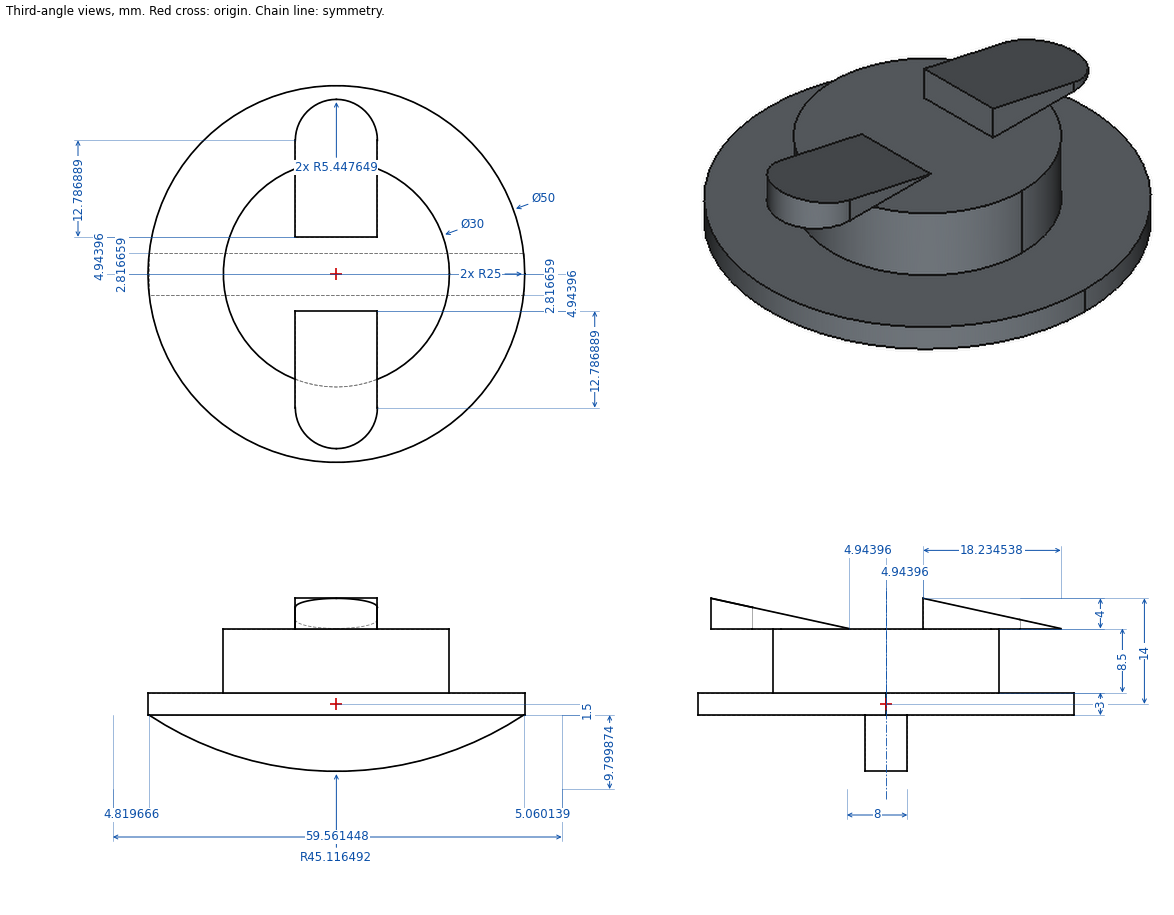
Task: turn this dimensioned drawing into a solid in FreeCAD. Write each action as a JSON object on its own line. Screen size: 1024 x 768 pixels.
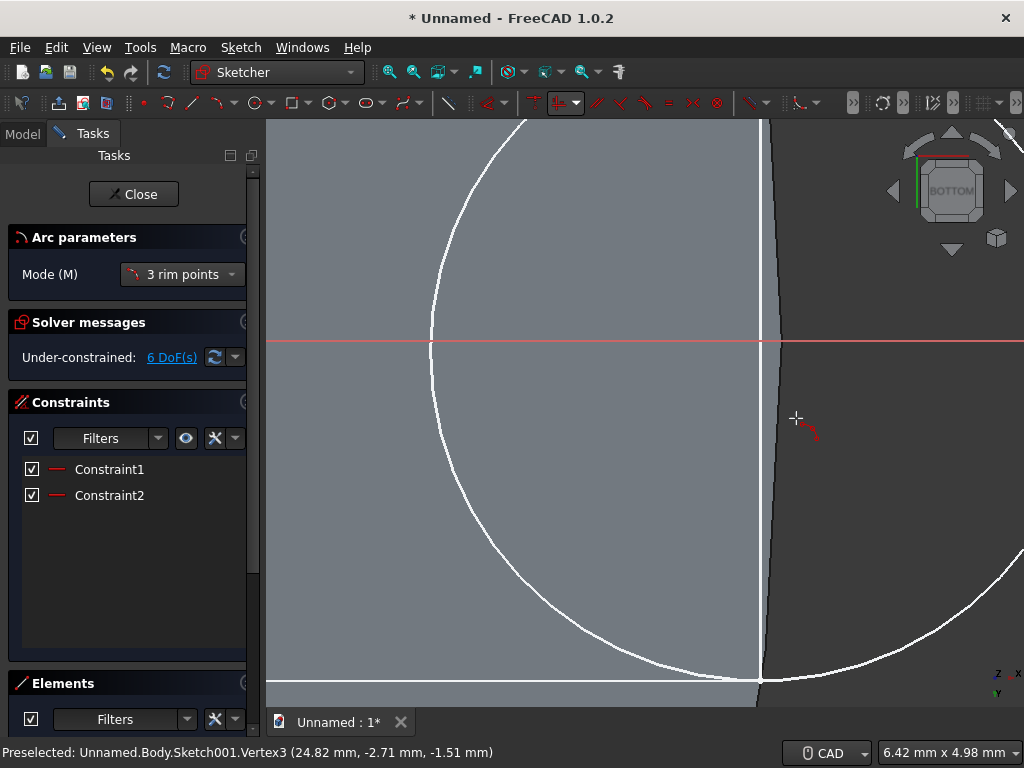
{"action": "left_click", "coordinate": [781, 408]}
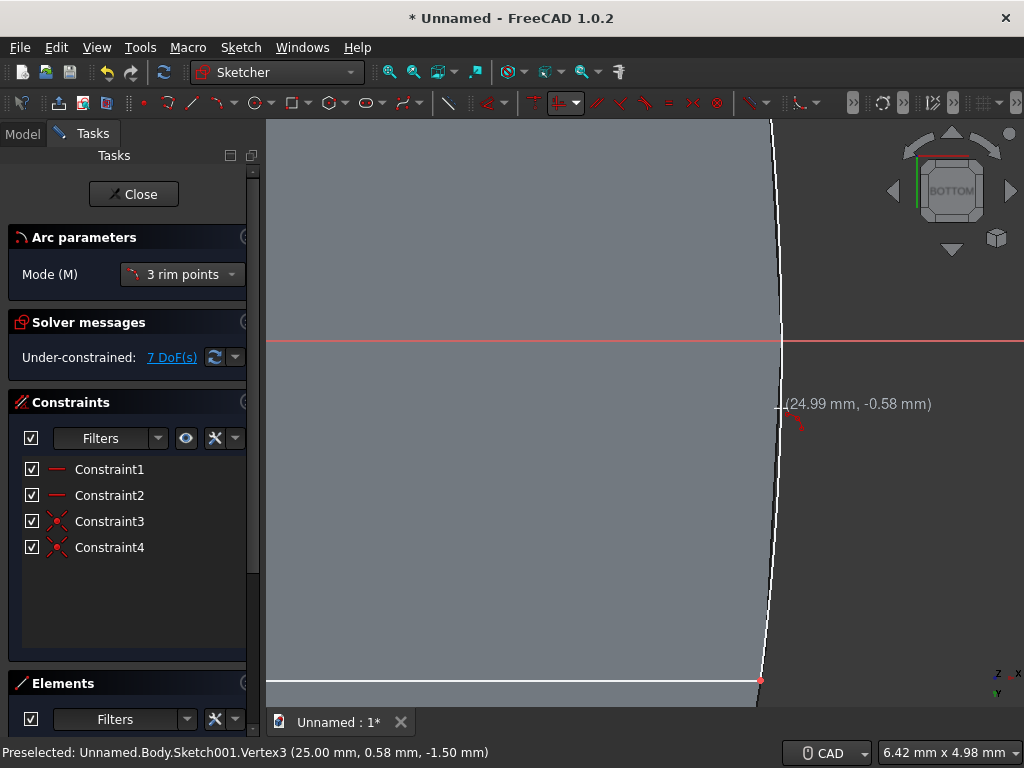
{"action": "scroll", "coordinate": [797, 419], "scroll_direction": "down", "scroll_amount": 13}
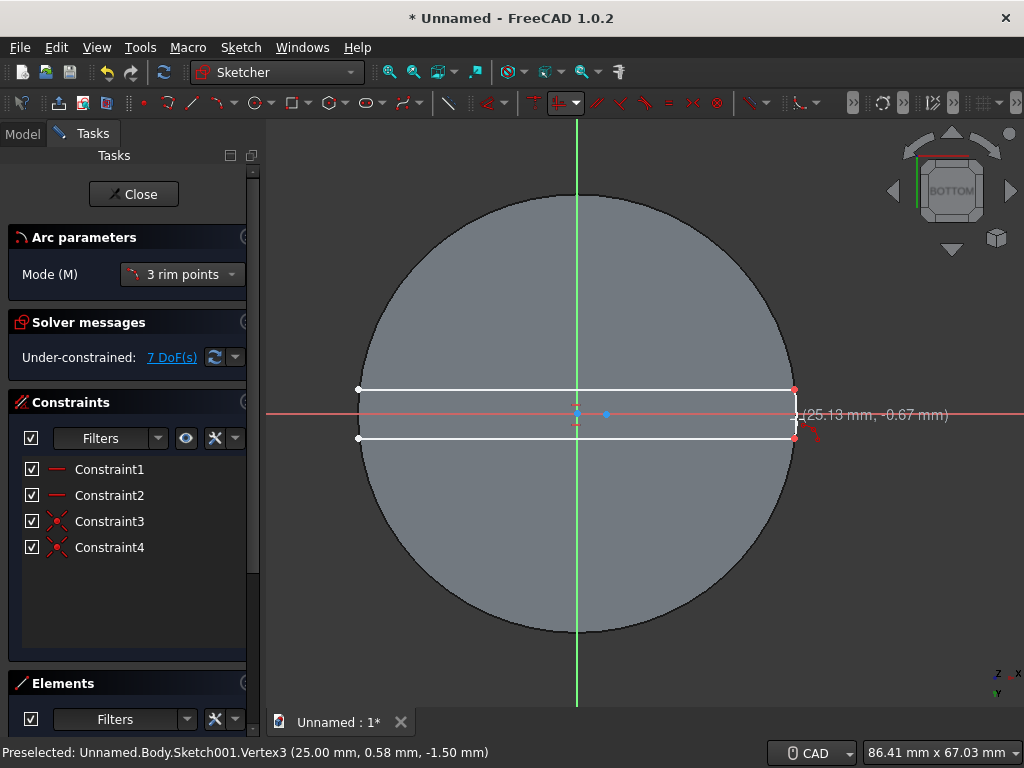
{"action": "left_click", "coordinate": [359, 390]}
{"action": "left_click", "coordinate": [359, 439]}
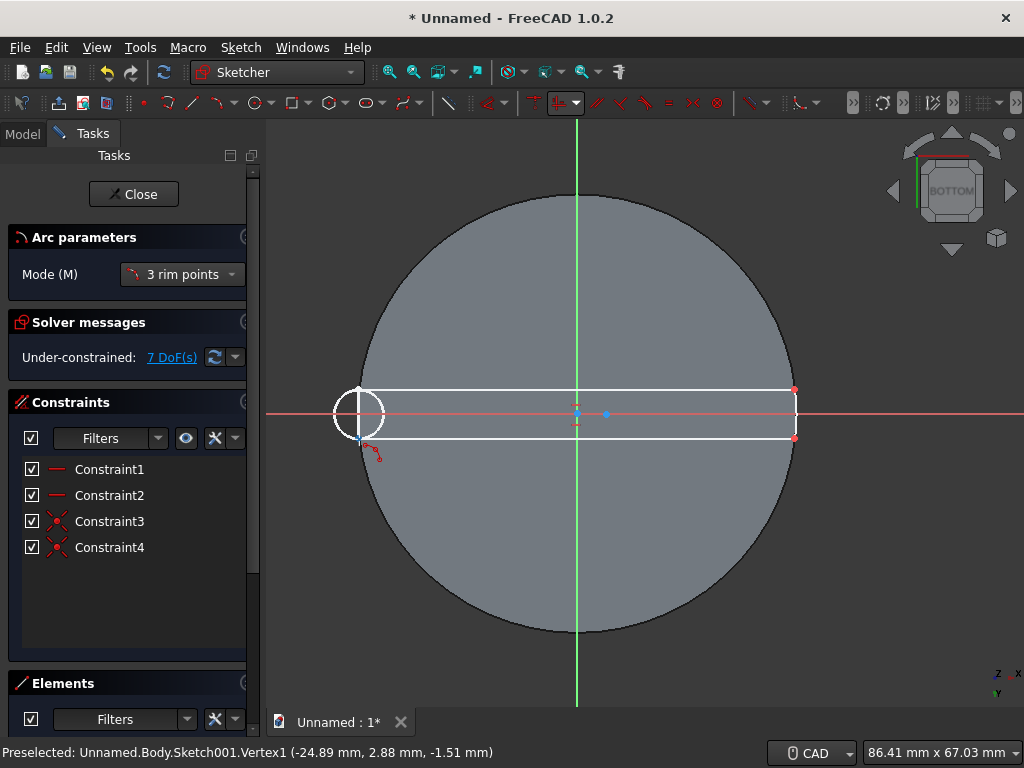
{"action": "scroll", "coordinate": [358, 409], "scroll_direction": "up", "scroll_amount": 13}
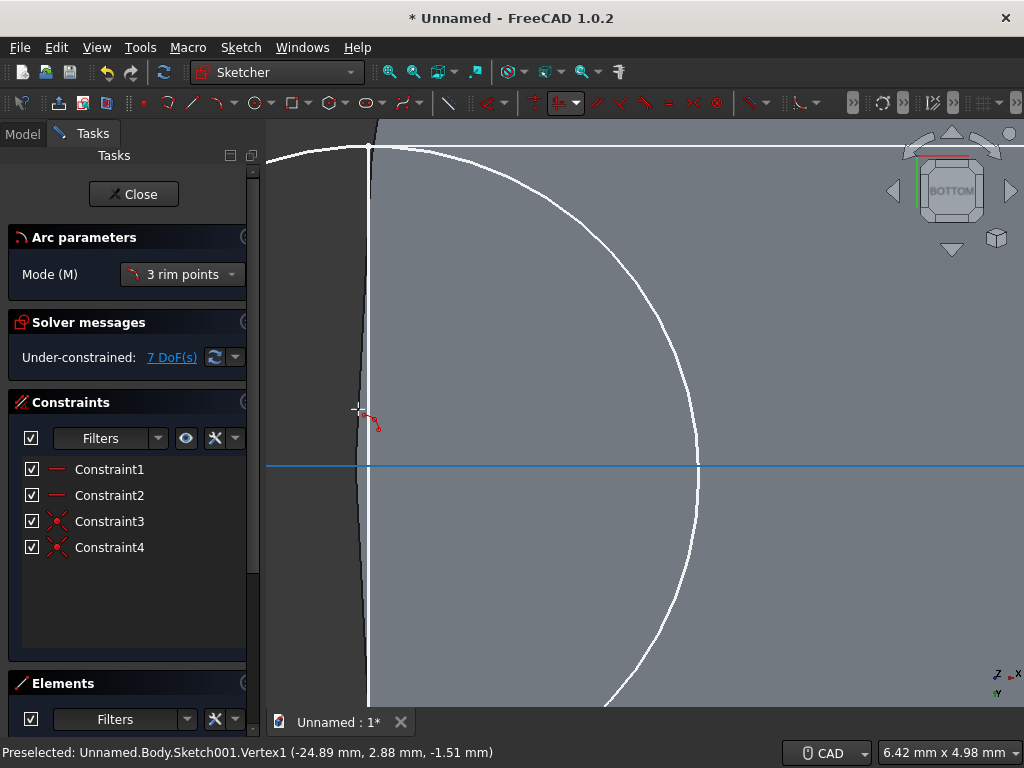
{"action": "left_click", "coordinate": [356, 399]}
{"action": "key", "text": "Escape"}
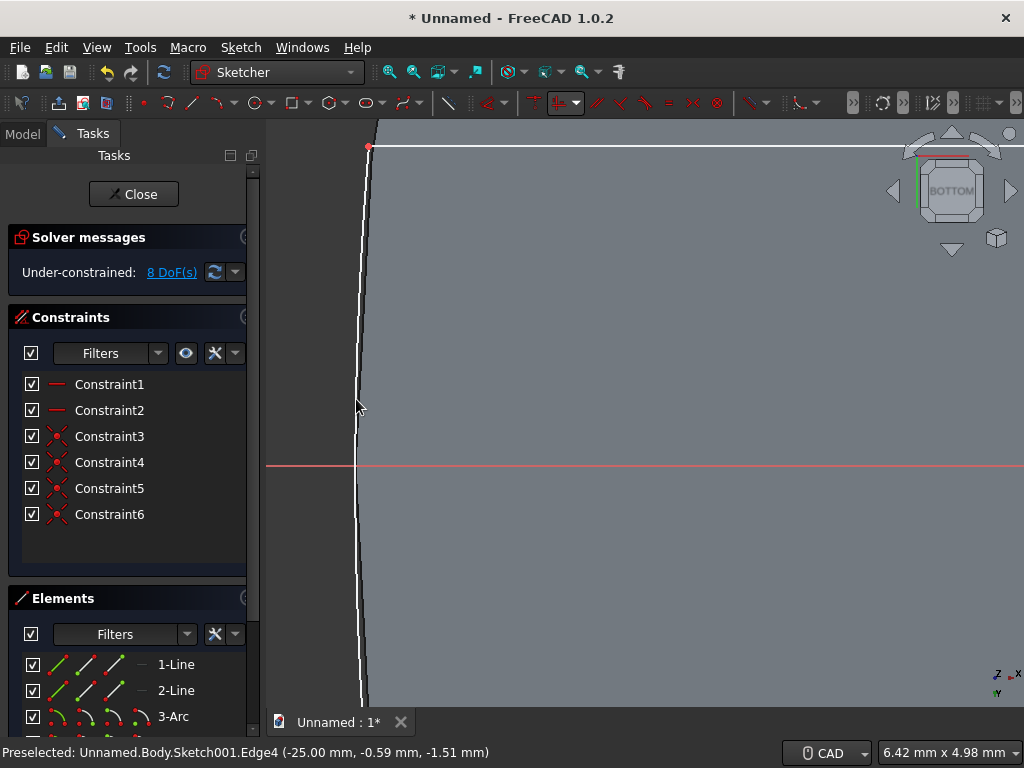
{"action": "scroll", "coordinate": [357, 409], "scroll_direction": "down", "scroll_amount": 13}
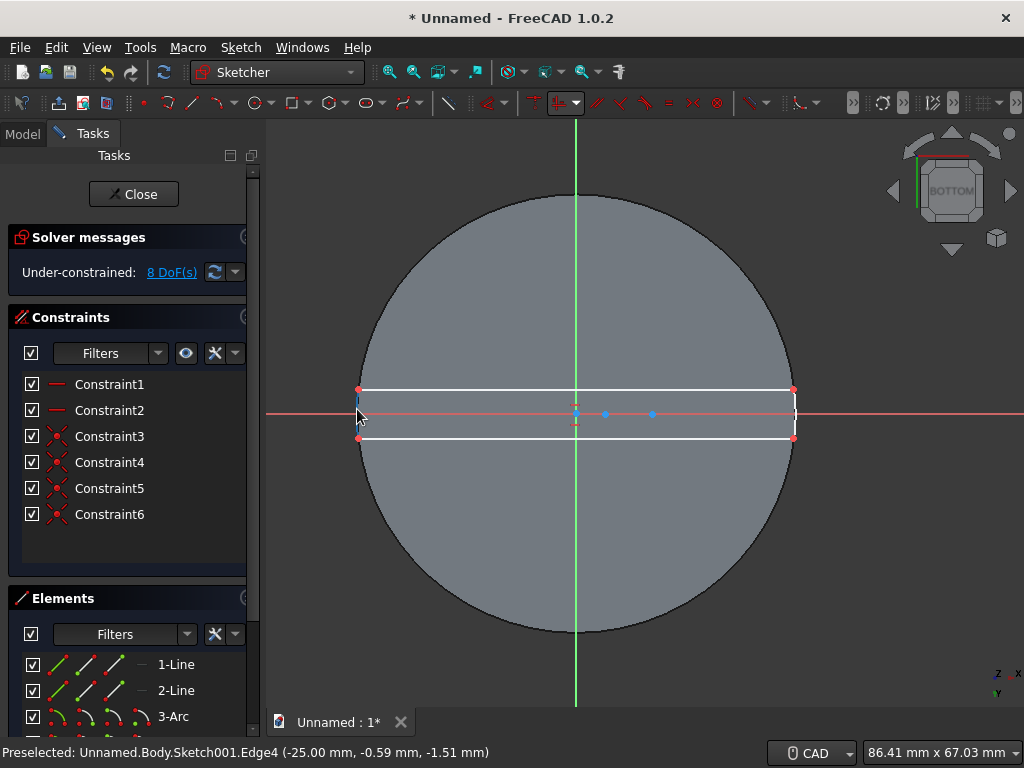
{"action": "scroll", "coordinate": [795, 424], "scroll_direction": "up", "scroll_amount": 2}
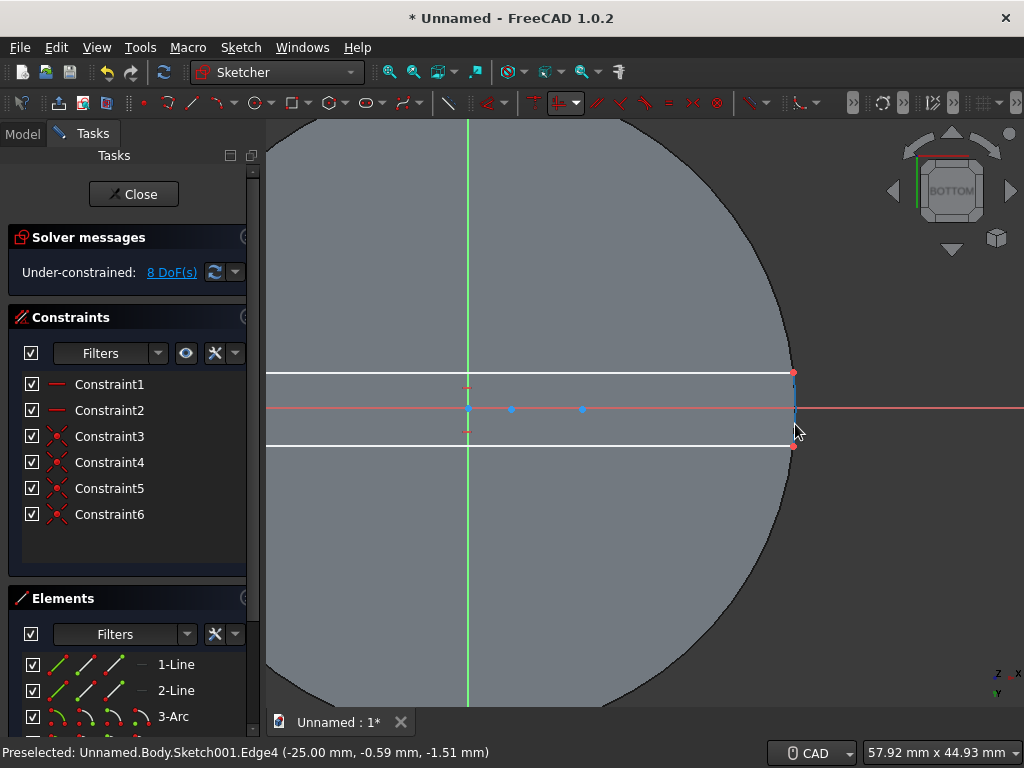
{"action": "left_click", "coordinate": [795, 424]}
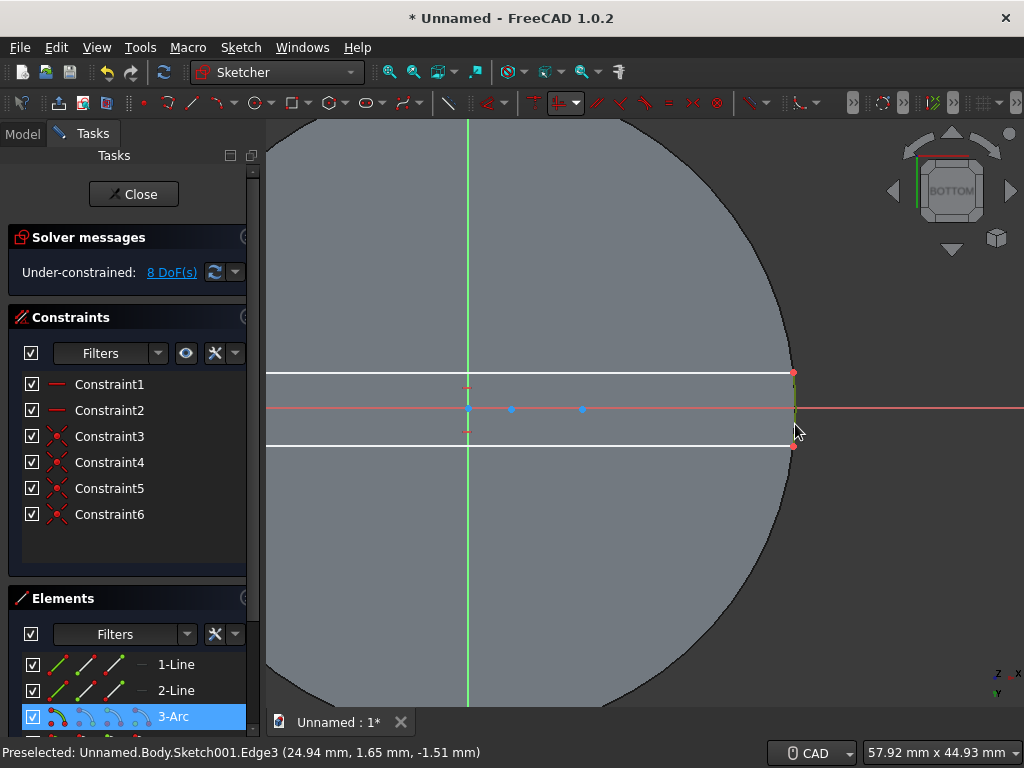
{"action": "scroll", "coordinate": [796, 422], "scroll_direction": "down", "scroll_amount": 2}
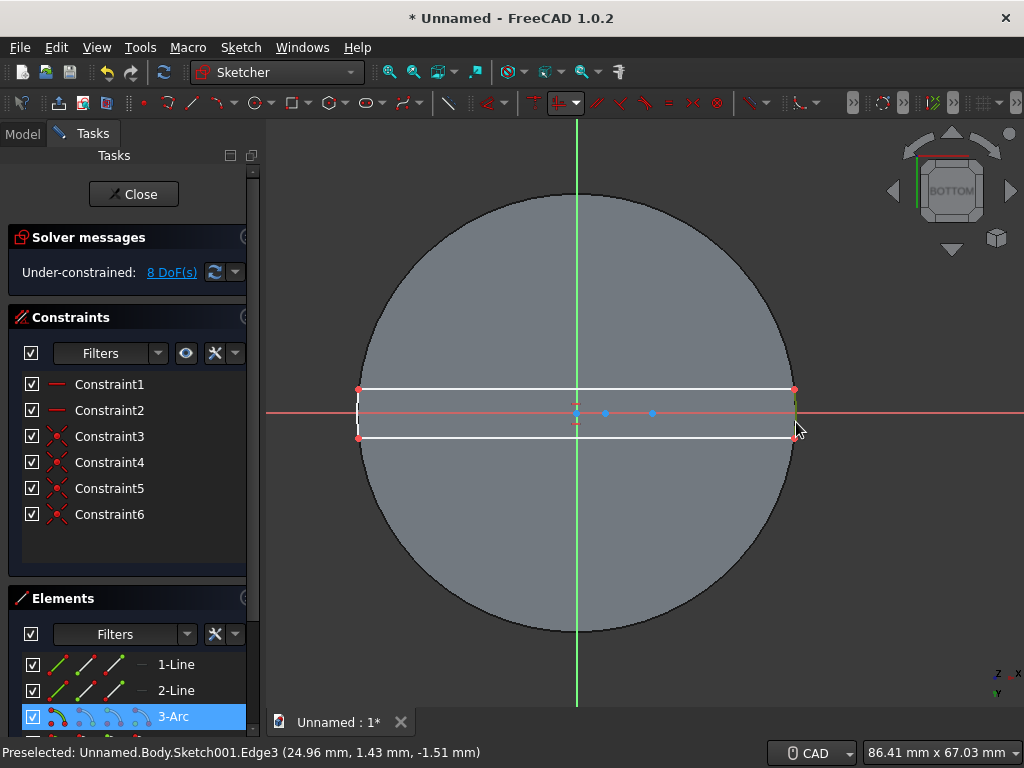
{"action": "scroll", "coordinate": [357, 404], "scroll_direction": "up", "scroll_amount": 3}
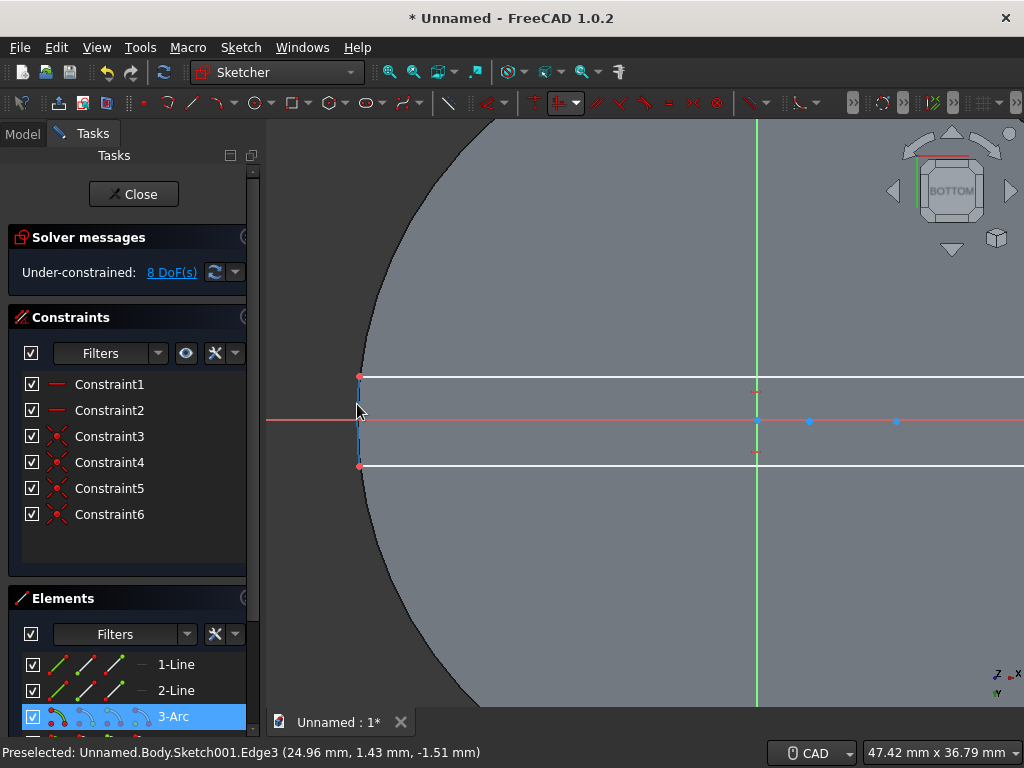
{"action": "left_click", "coordinate": [358, 404]}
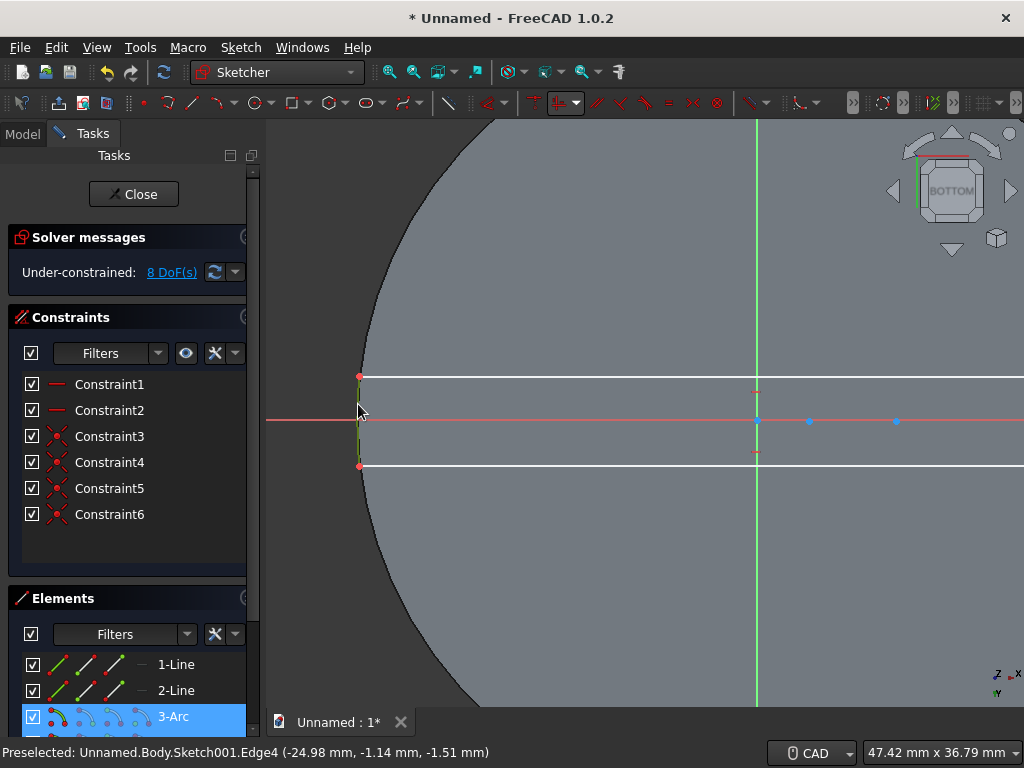
{"action": "left_click", "coordinate": [534, 104]}